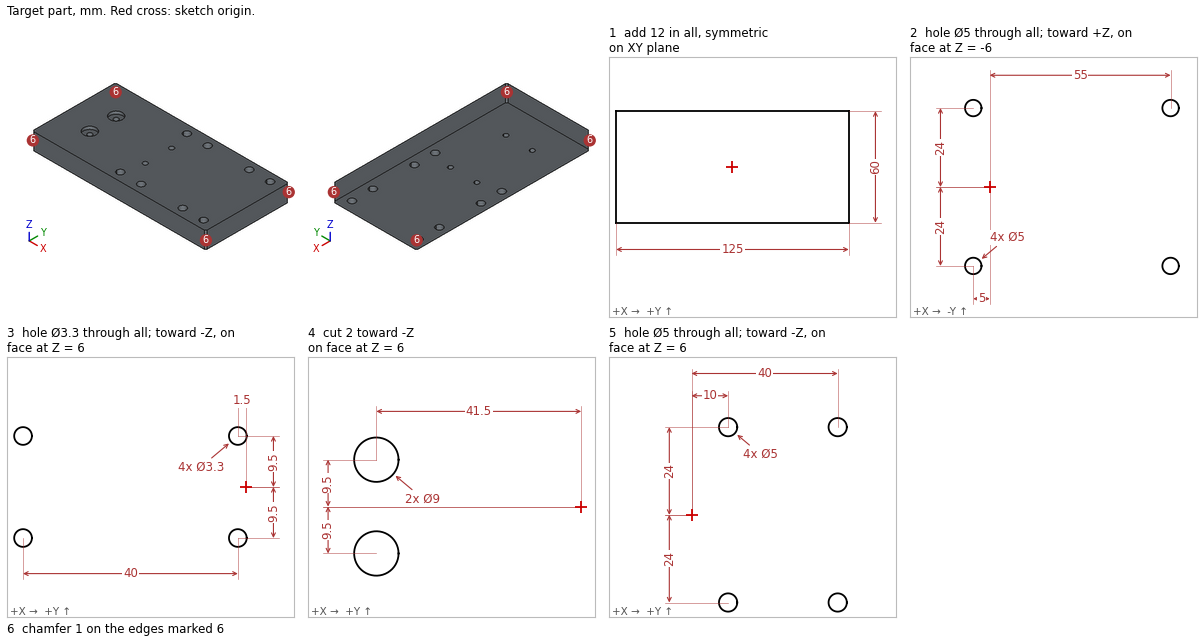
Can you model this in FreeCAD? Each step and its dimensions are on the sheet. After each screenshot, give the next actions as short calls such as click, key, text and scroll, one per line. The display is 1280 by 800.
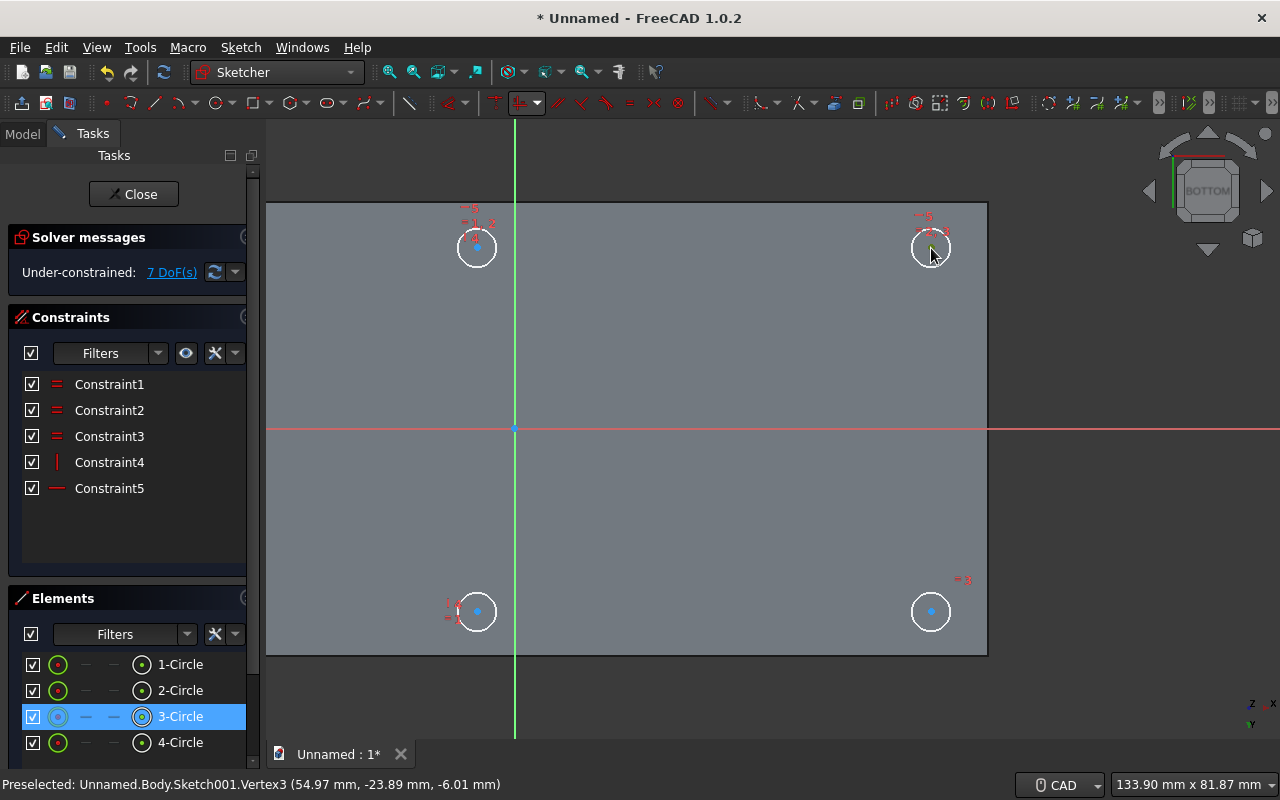
click(931, 612)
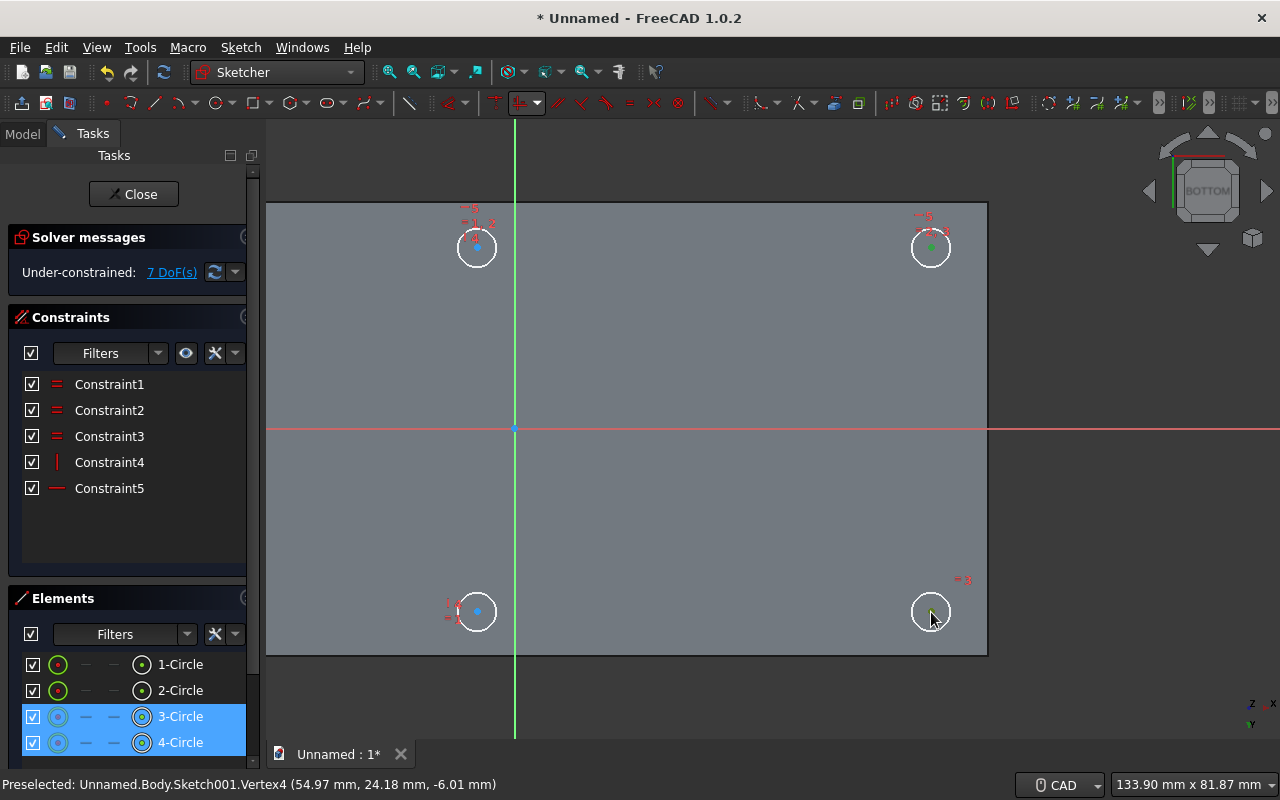
key(v)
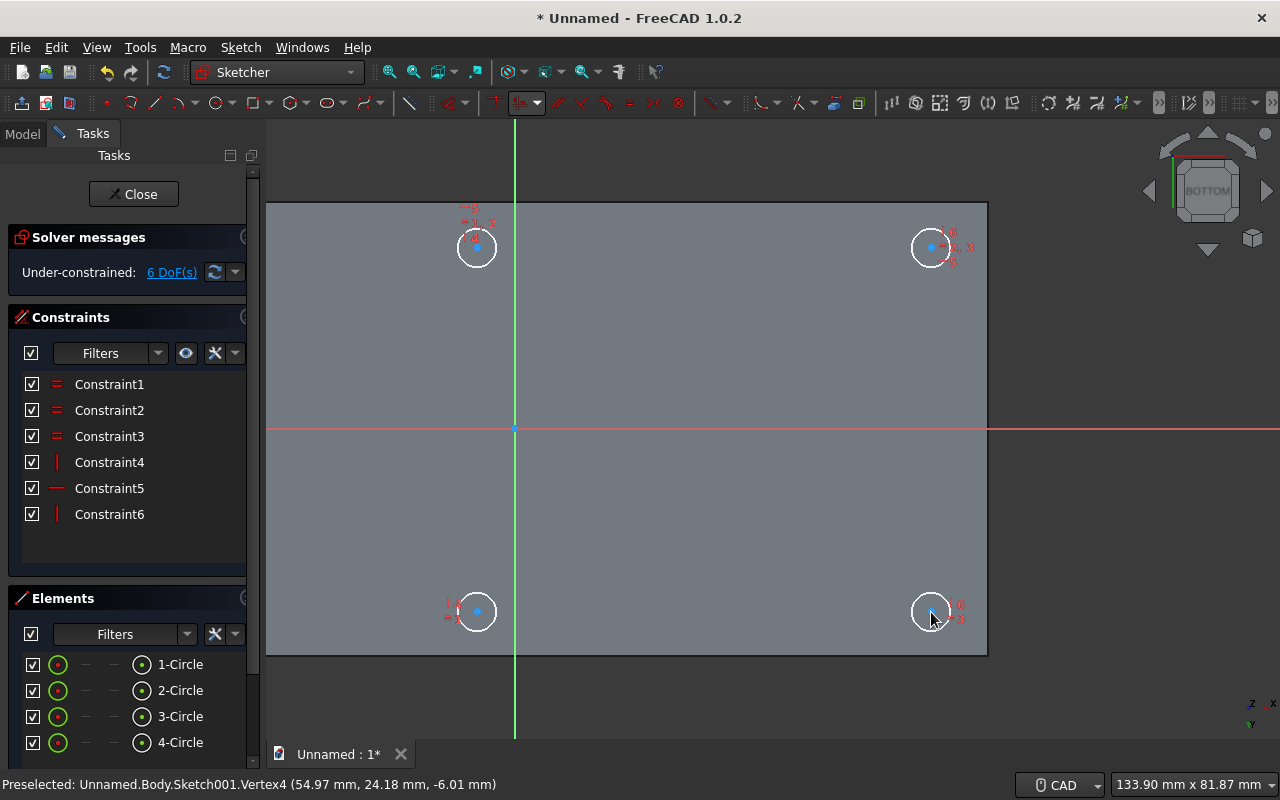
click(477, 612)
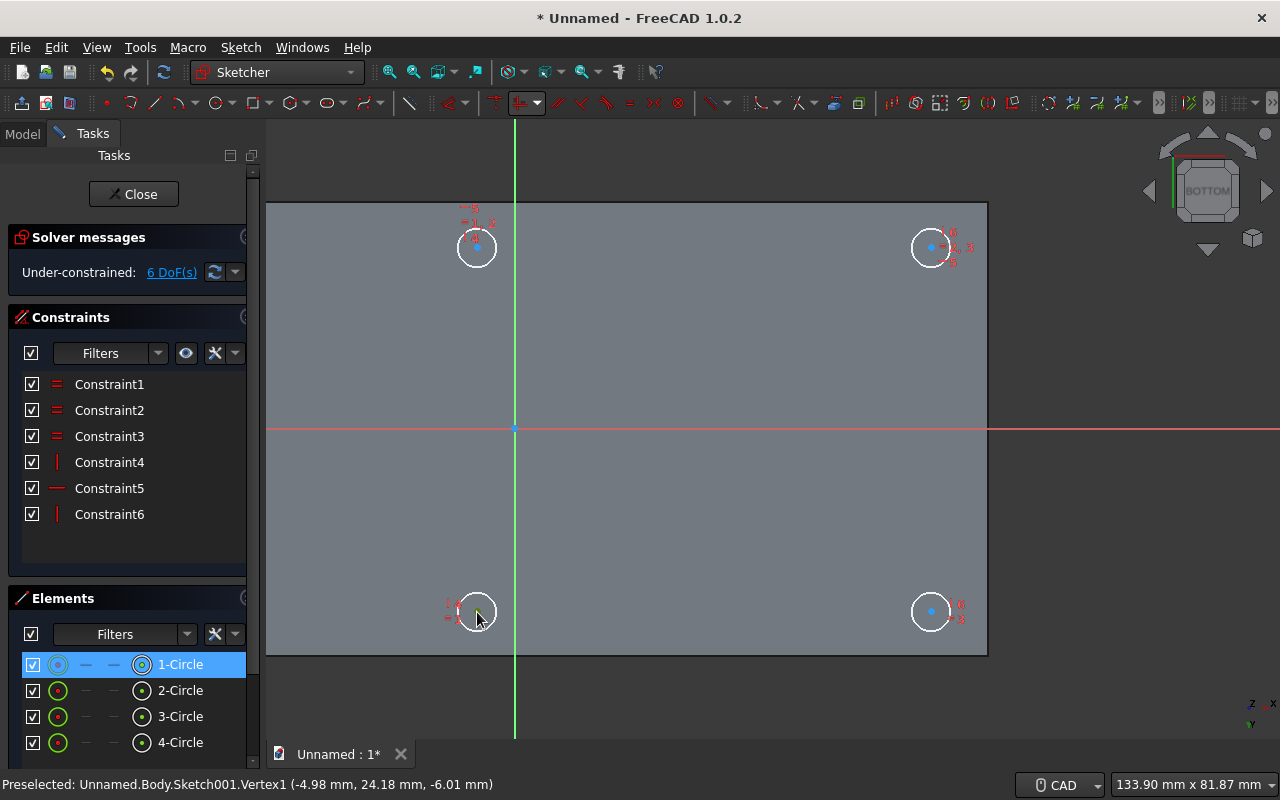
click(931, 612)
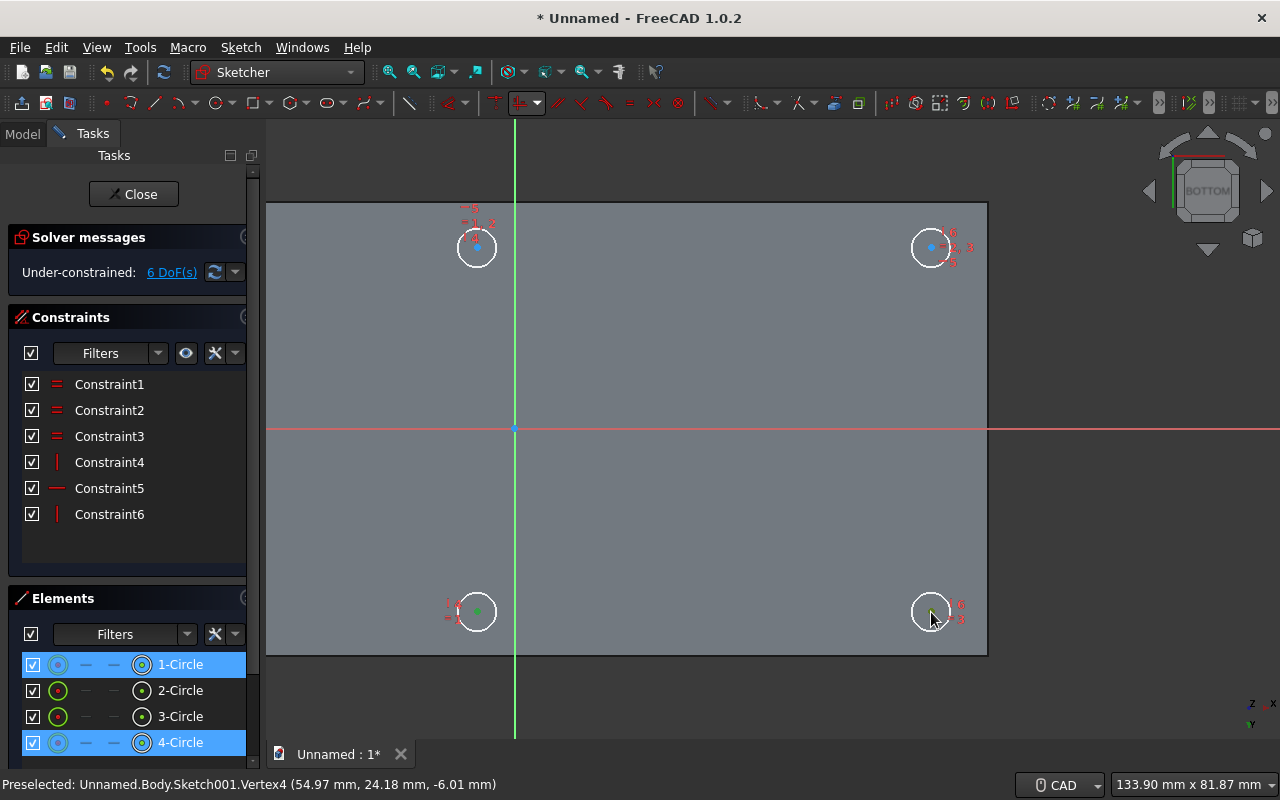
key(h)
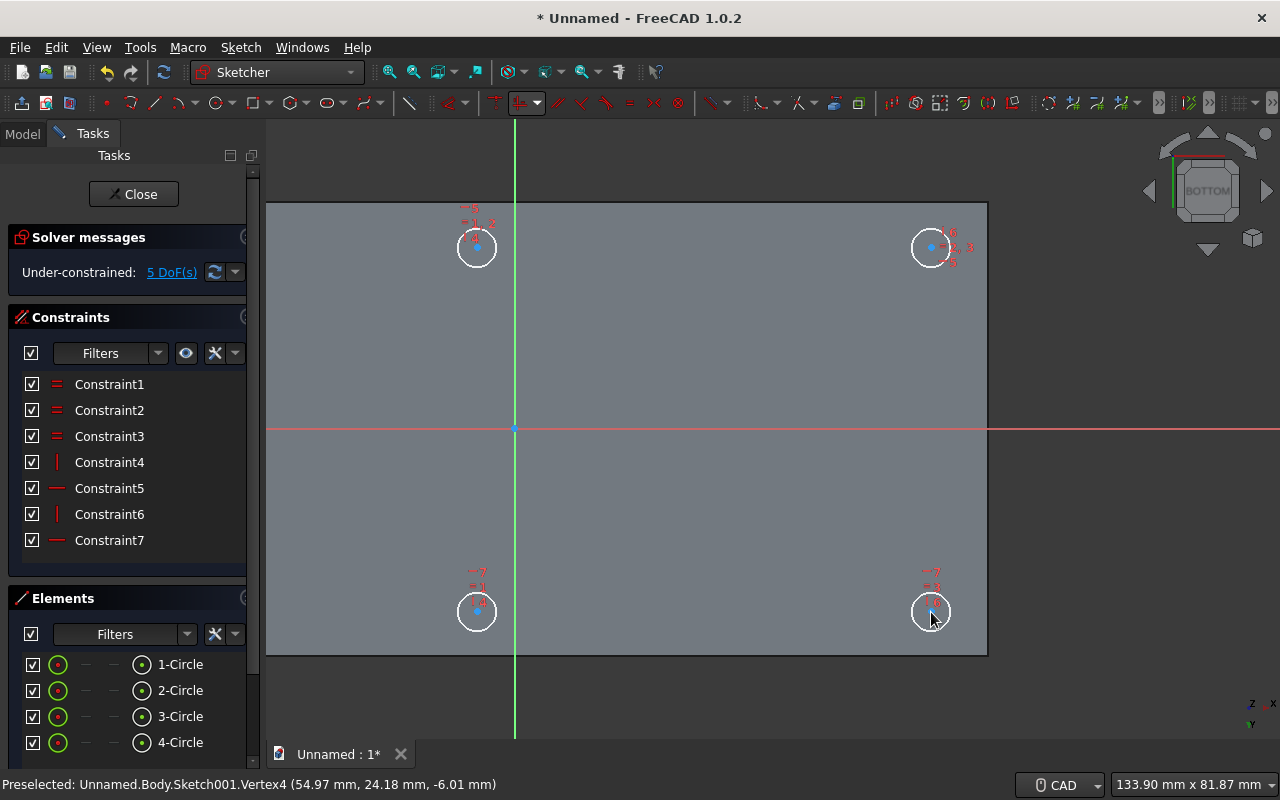
click(490, 598)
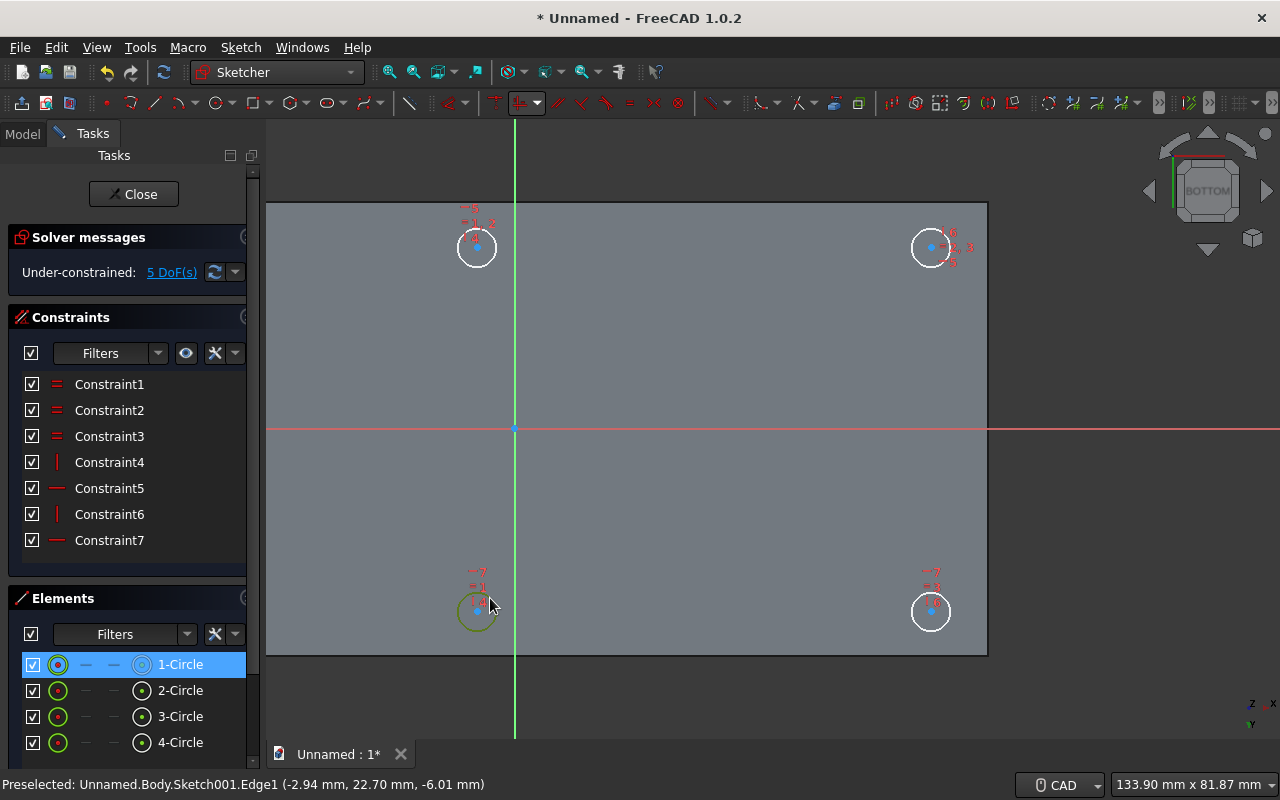
key(k)
key(o)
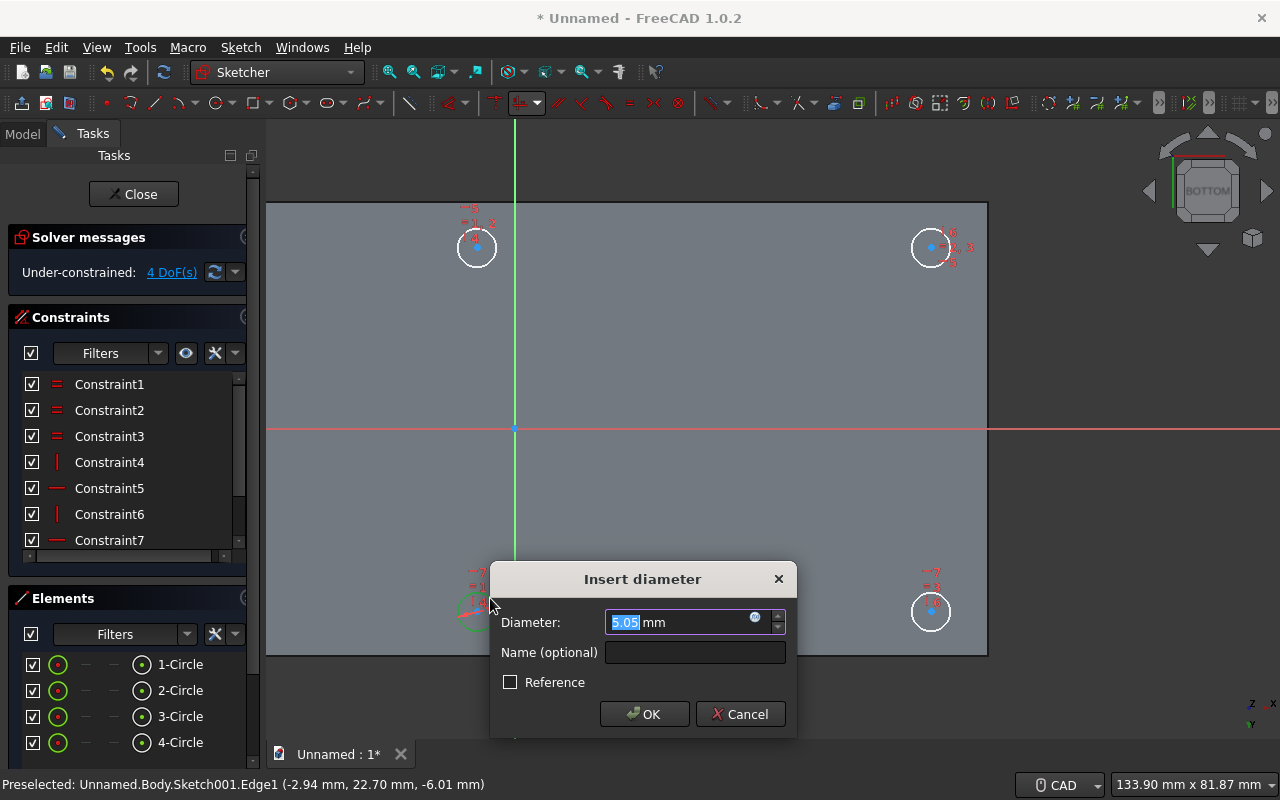
text(5)
key(Return)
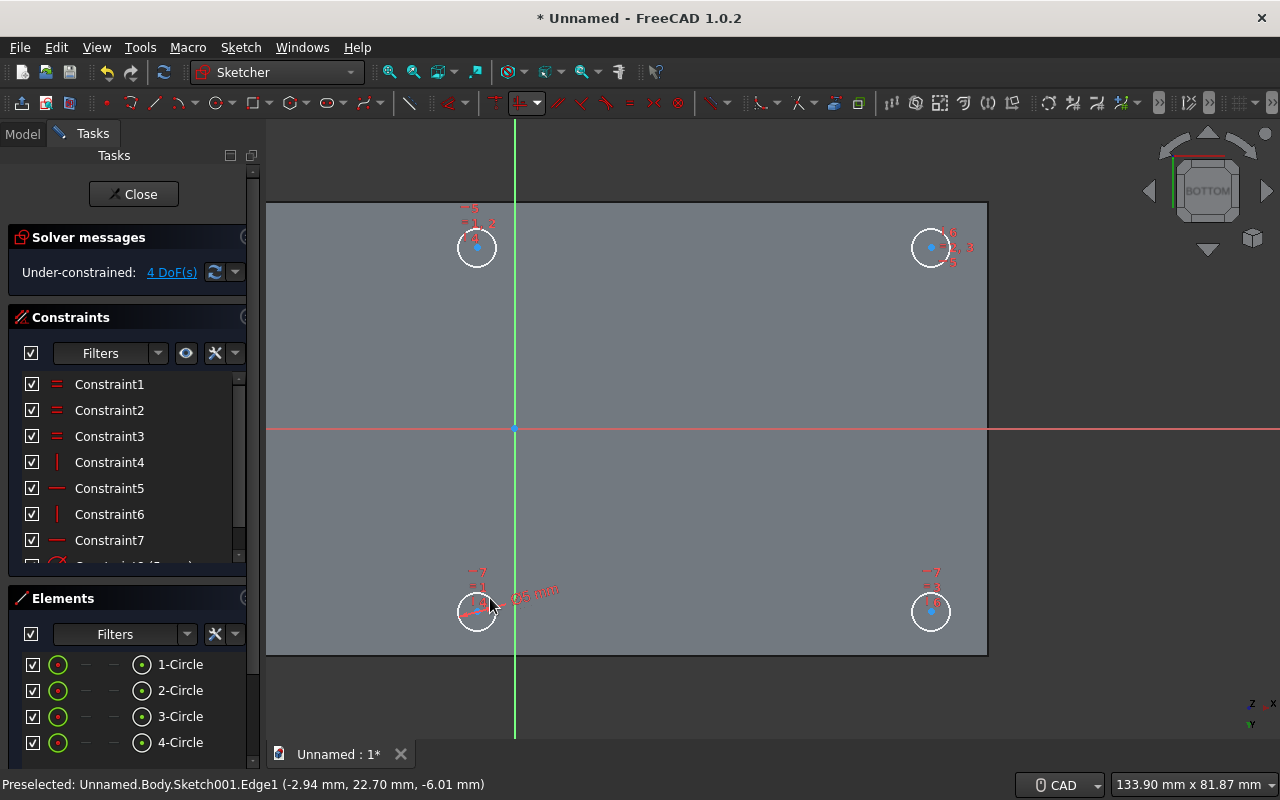
click(477, 612)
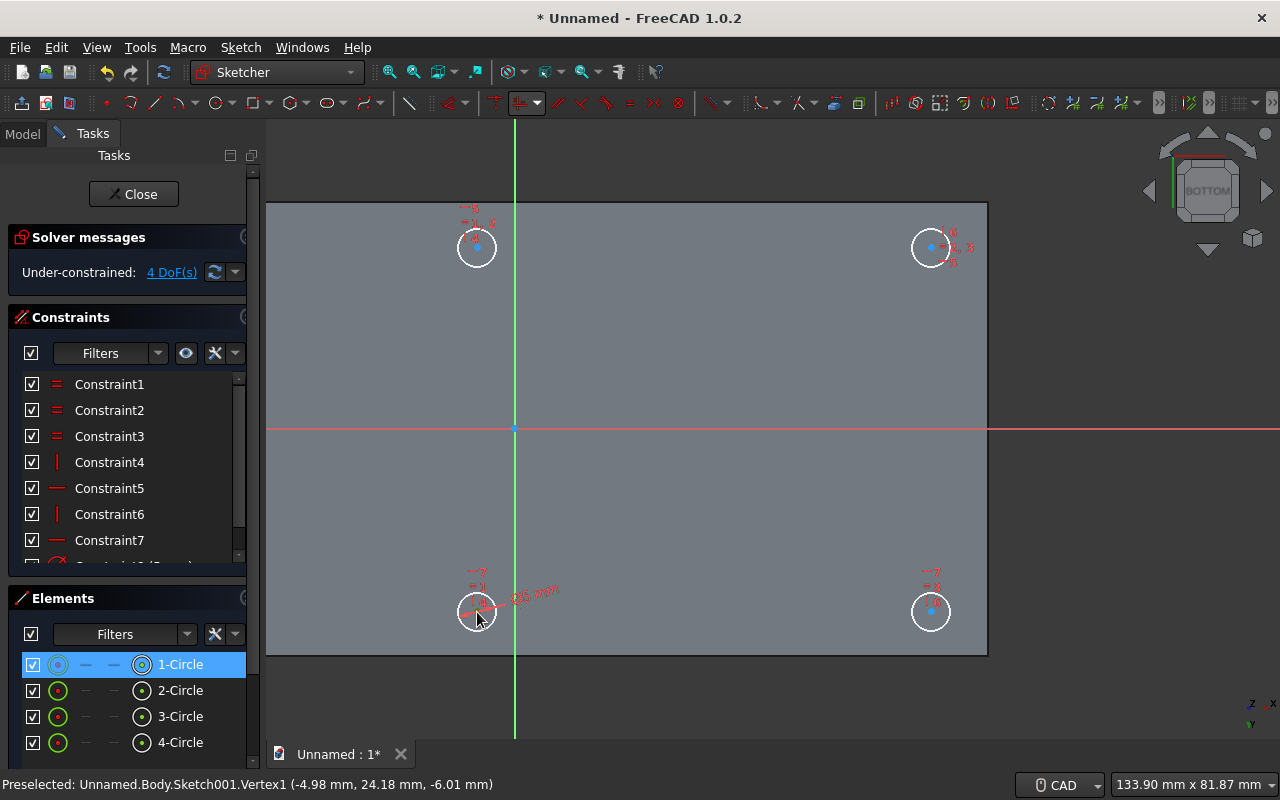
click(468, 104)